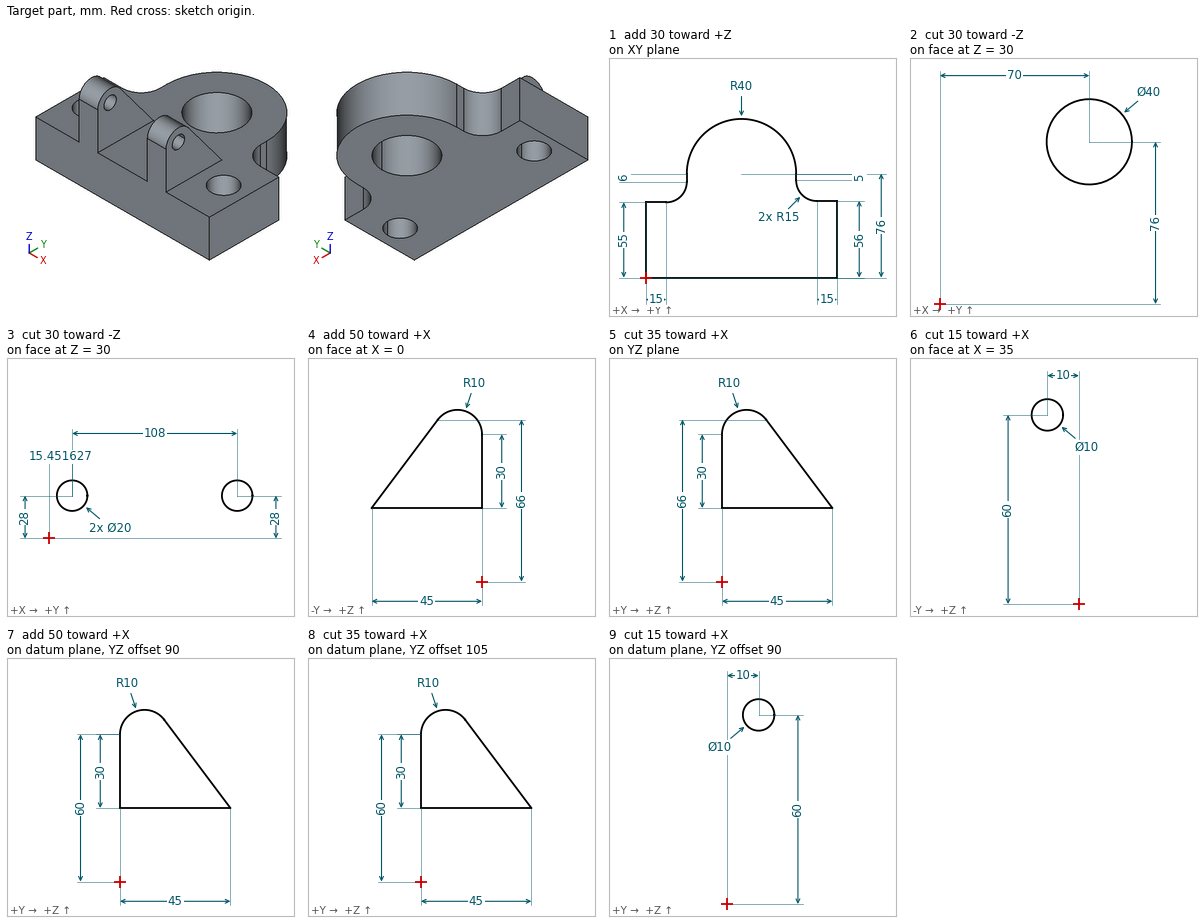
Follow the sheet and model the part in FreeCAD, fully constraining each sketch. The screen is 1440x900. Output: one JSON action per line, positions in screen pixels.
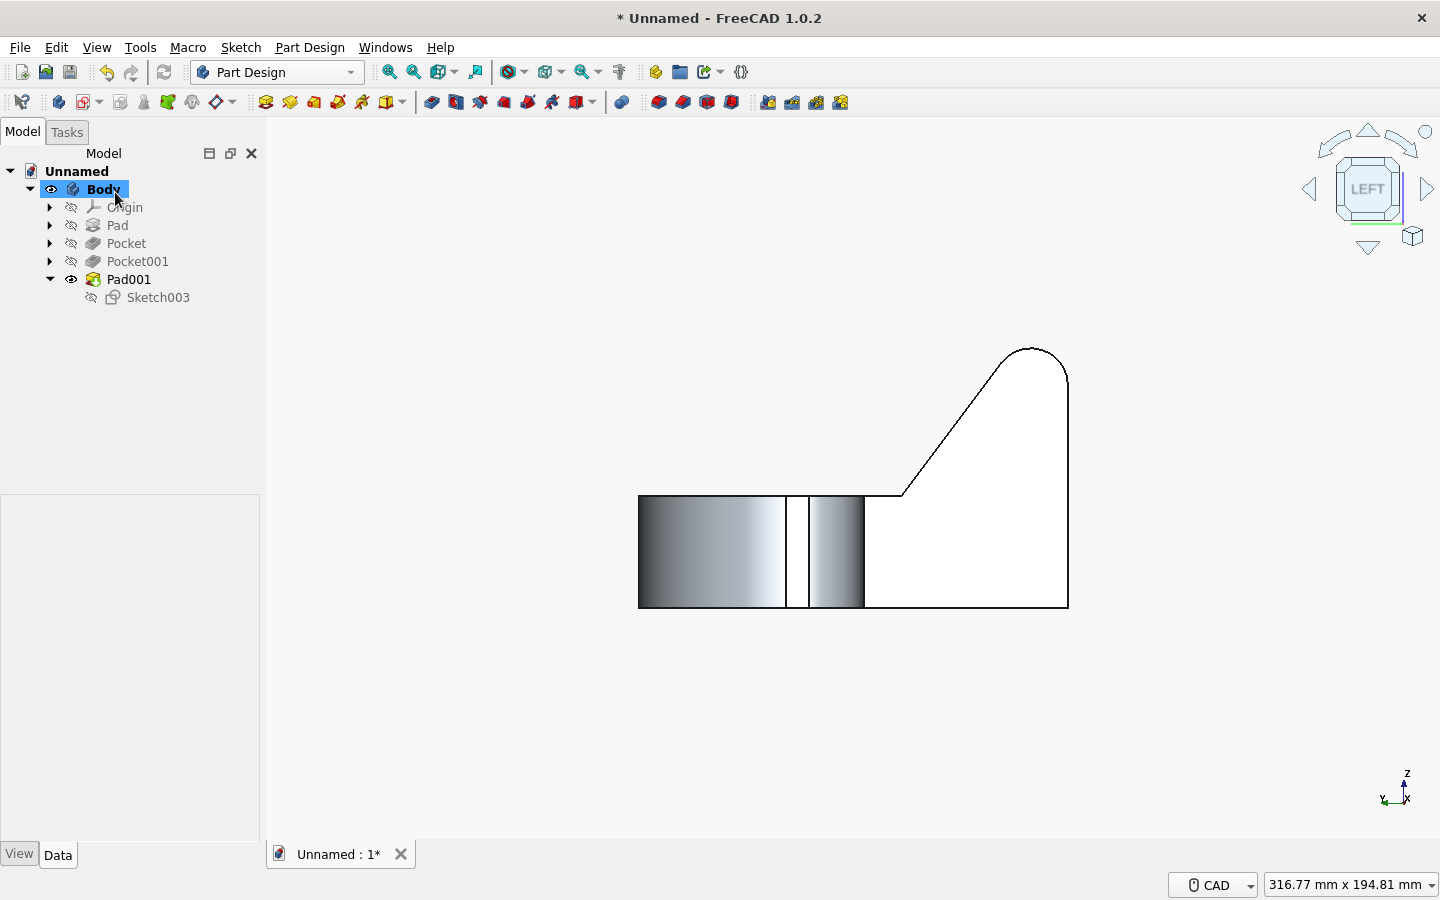
{"action": "left_click", "coordinate": [84, 102]}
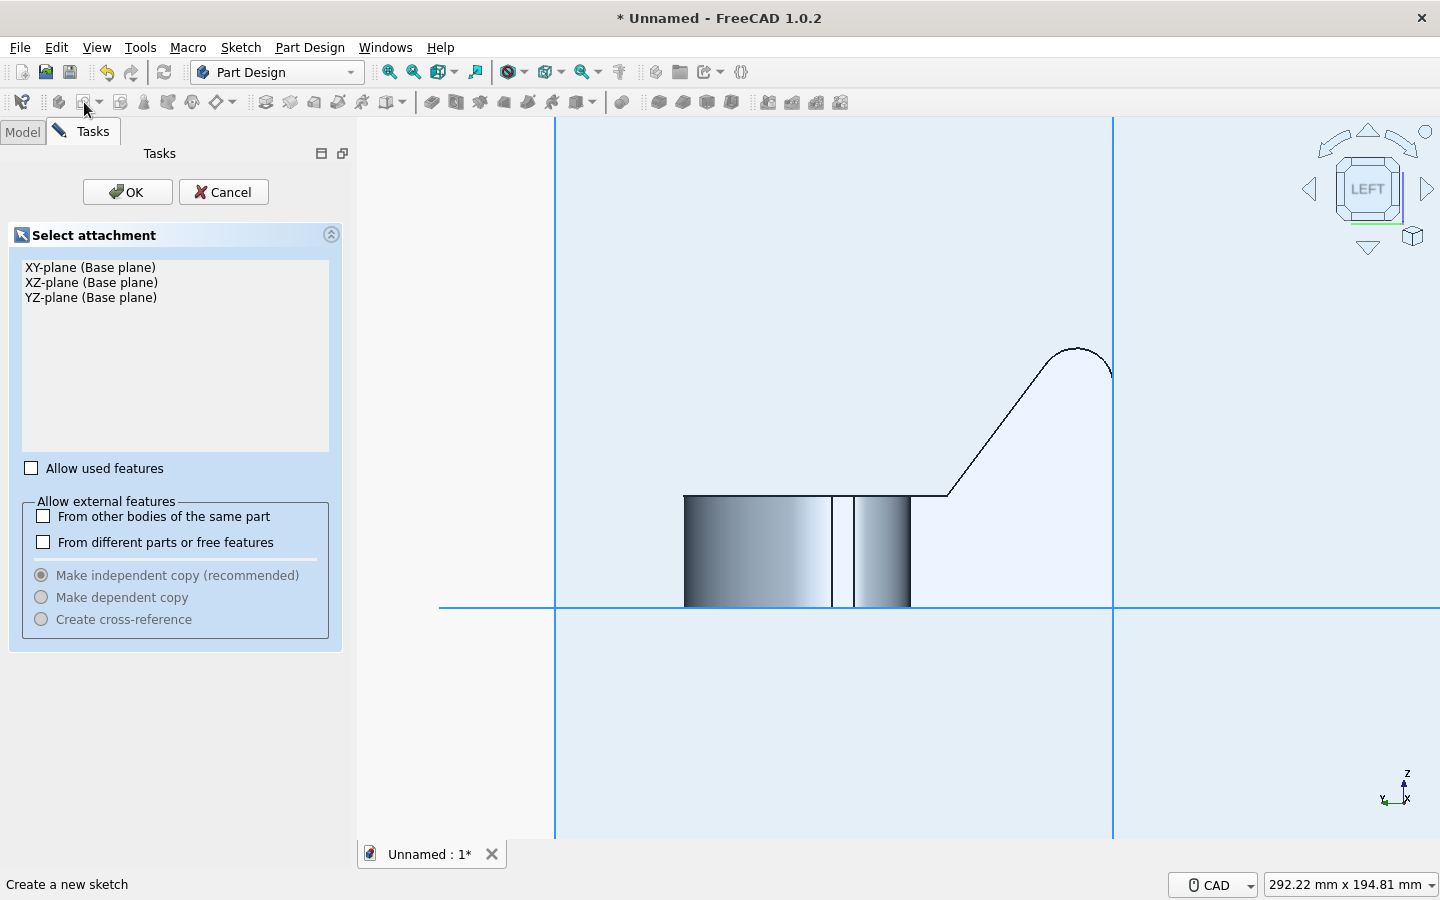
{"action": "left_click", "coordinate": [82, 298]}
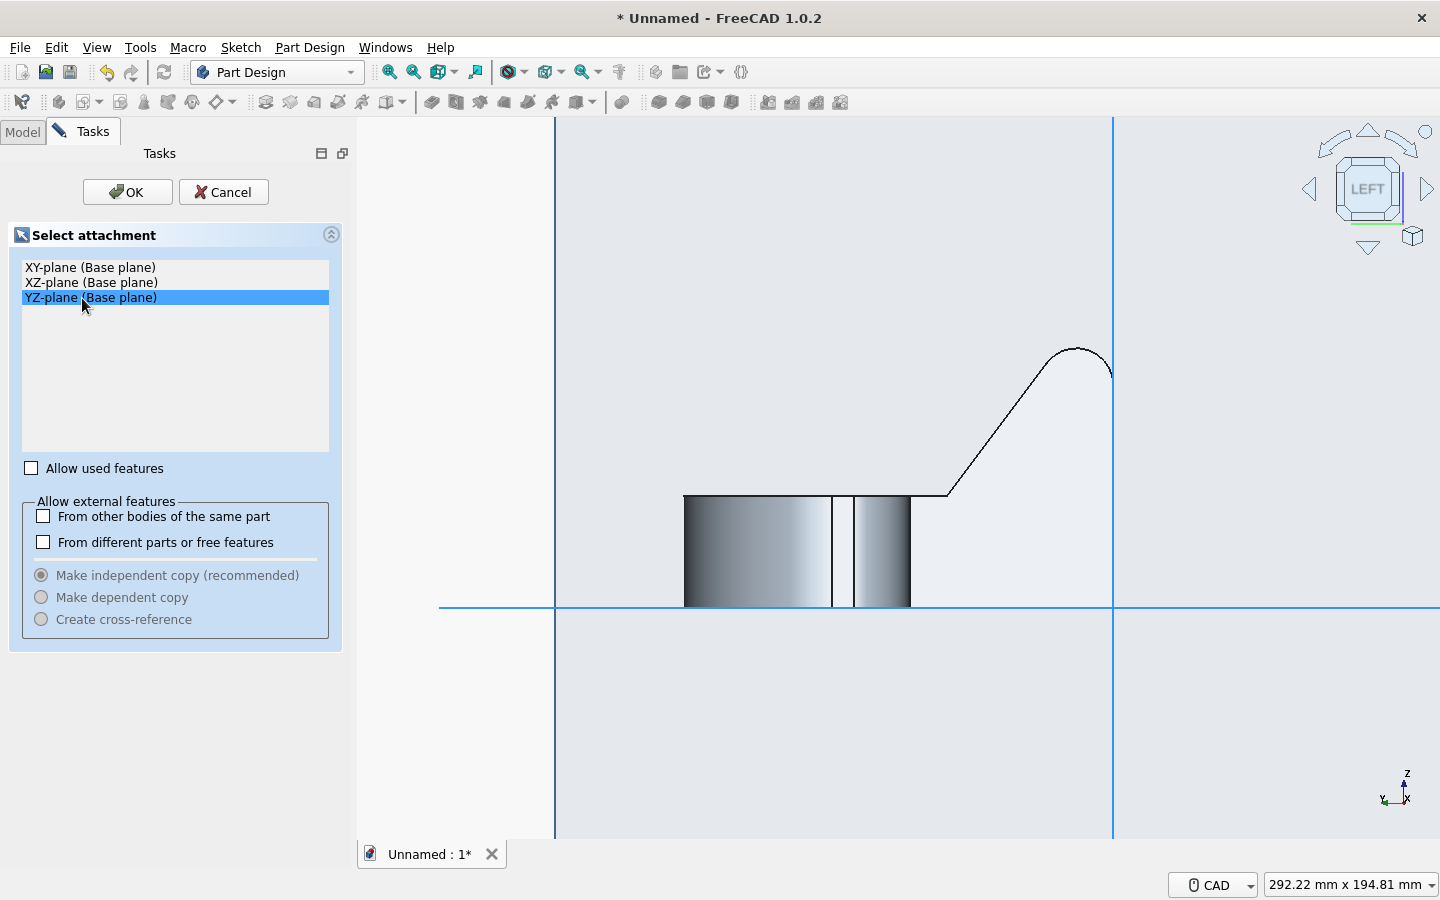
{"action": "left_click", "coordinate": [128, 192]}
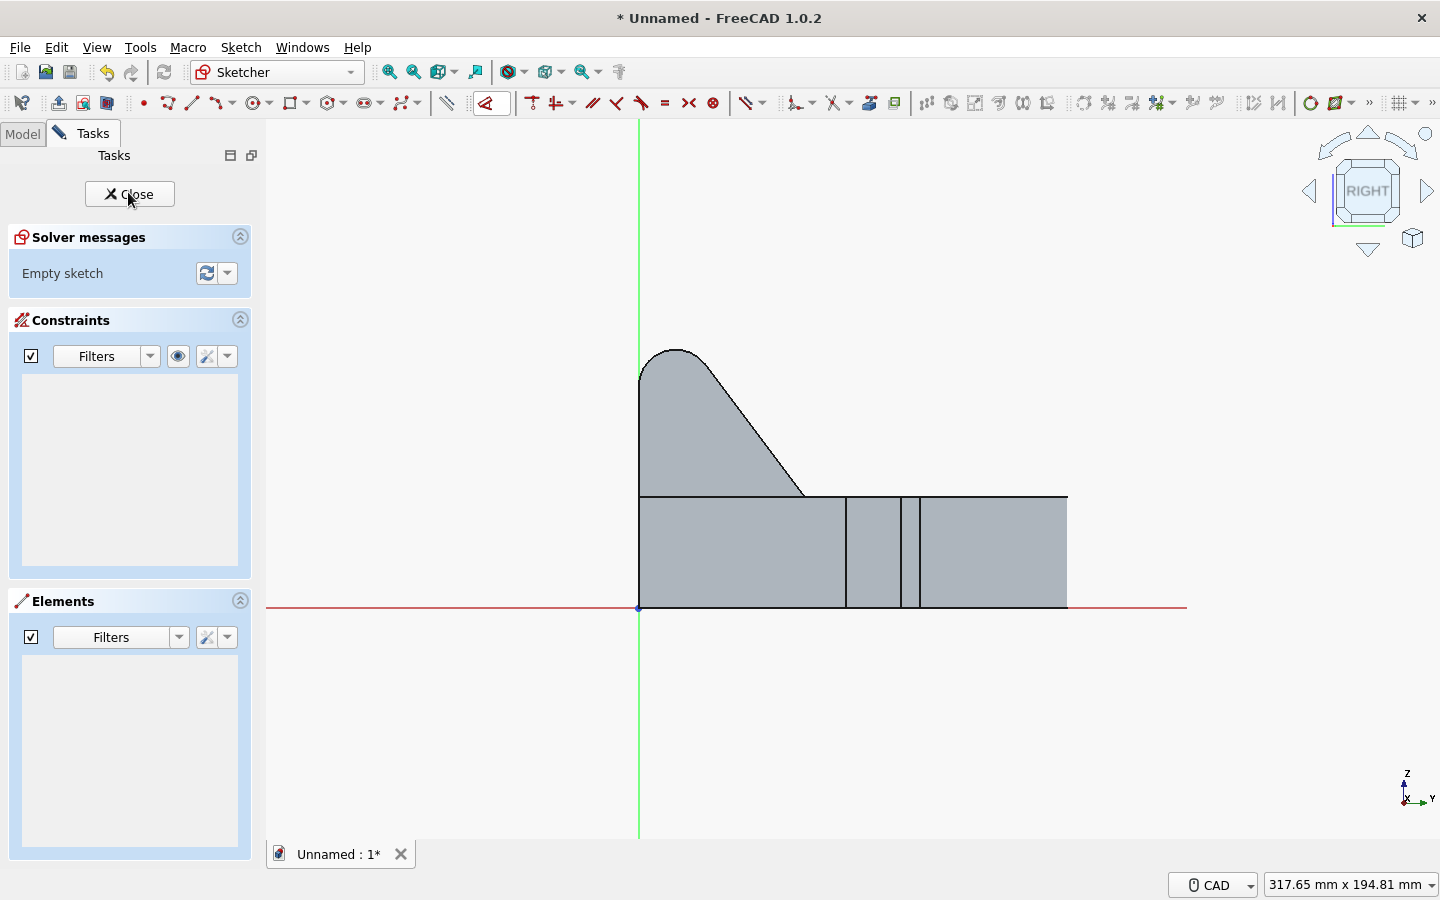
{"action": "key", "text": "q s"}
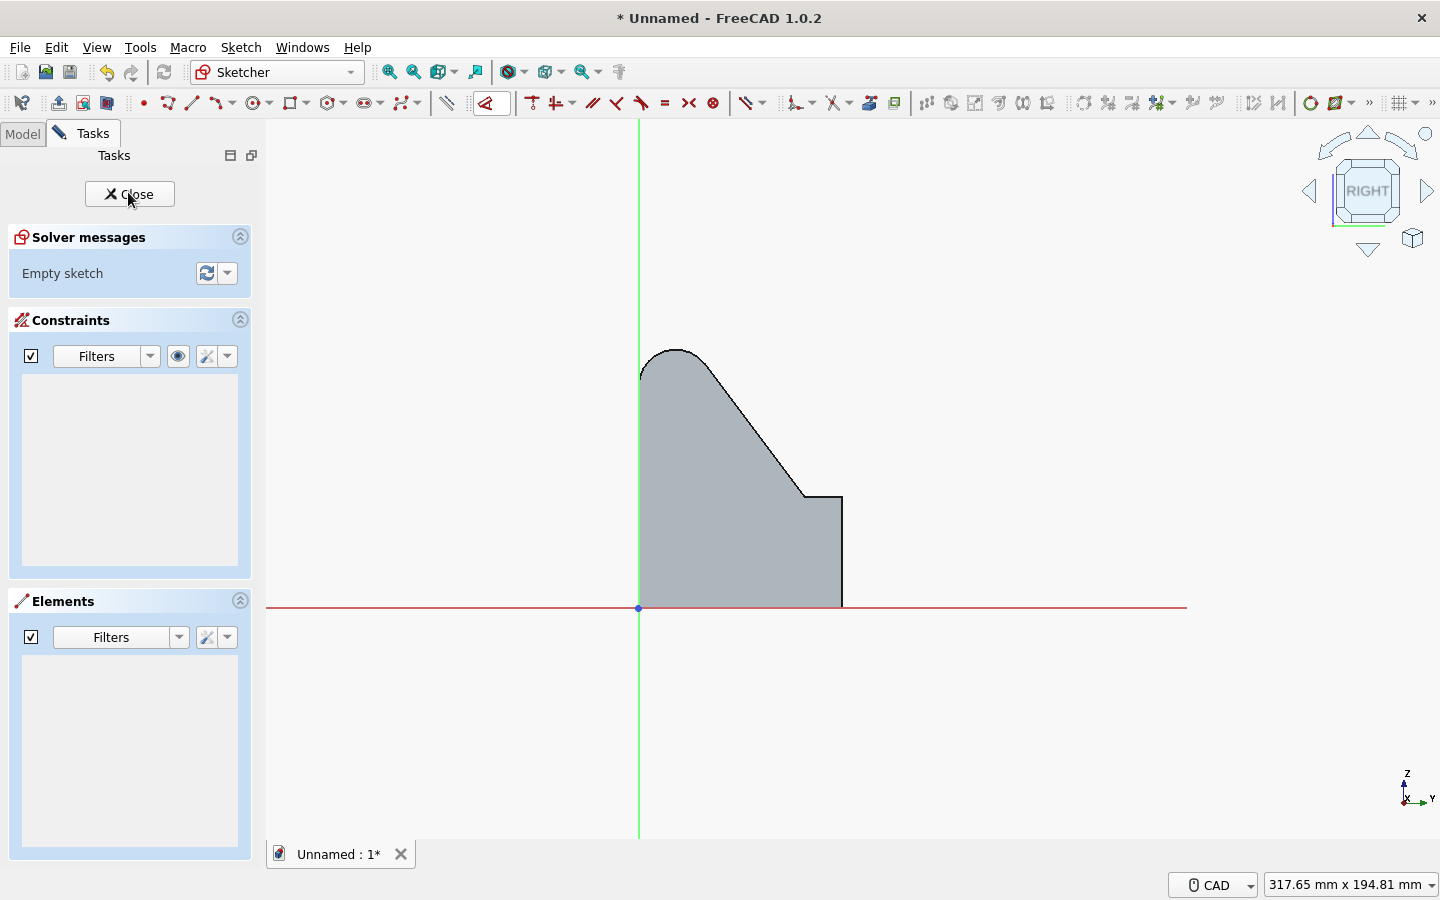
{"action": "scroll", "coordinate": [646, 481], "scroll_direction": "up", "scroll_amount": 3}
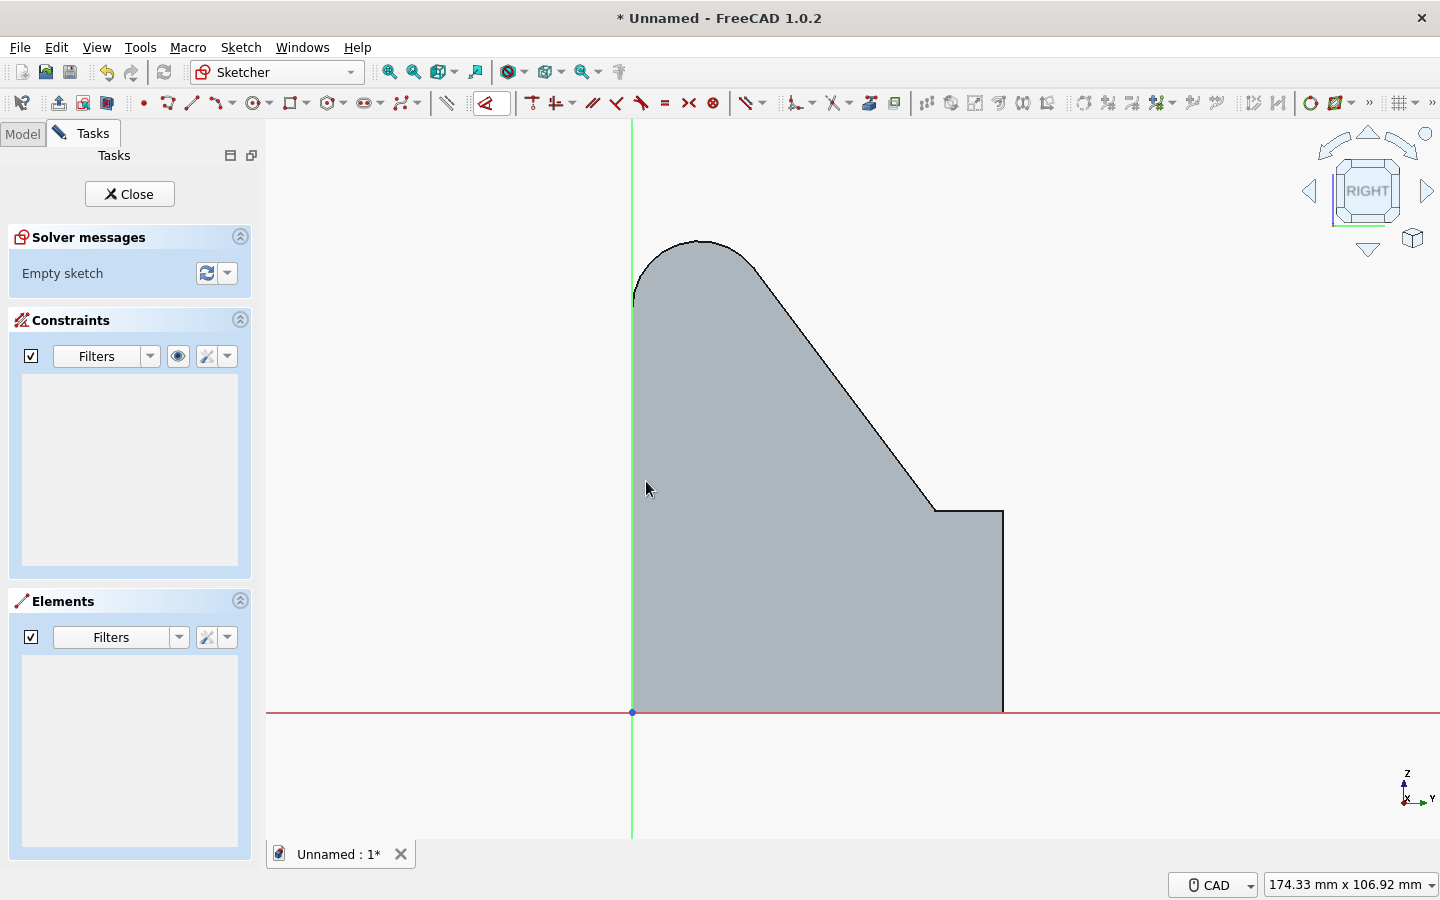
{"action": "key", "text": "g m"}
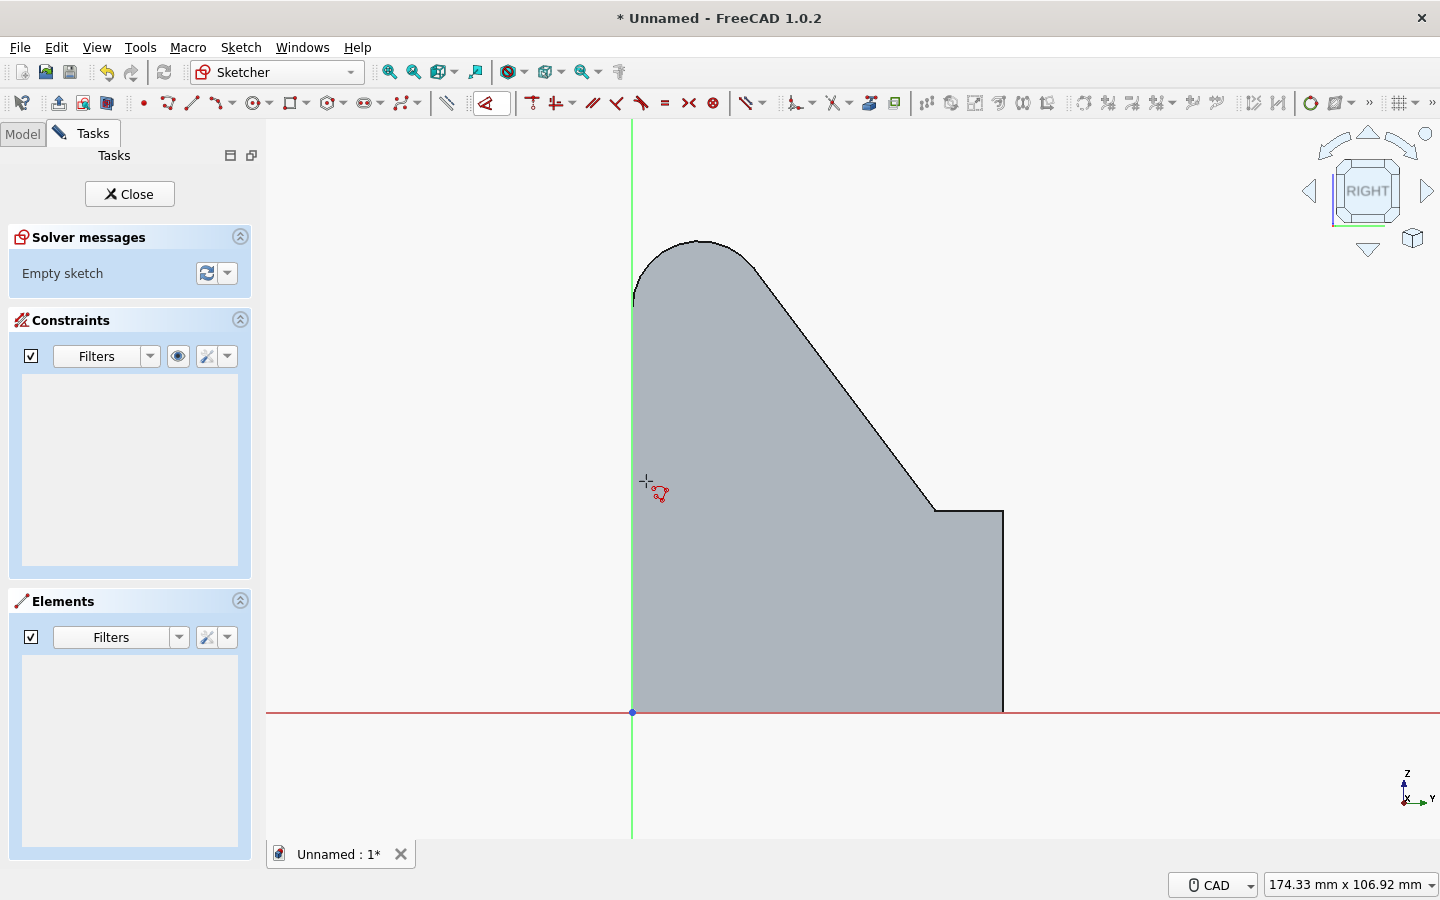
{"action": "left_click", "coordinate": [754, 268]}
{"action": "left_click", "coordinate": [935, 511]}
{"action": "left_click", "coordinate": [632, 511]}
{"action": "left_click", "coordinate": [641, 308]}
{"action": "right_click", "coordinate": [641, 308]}